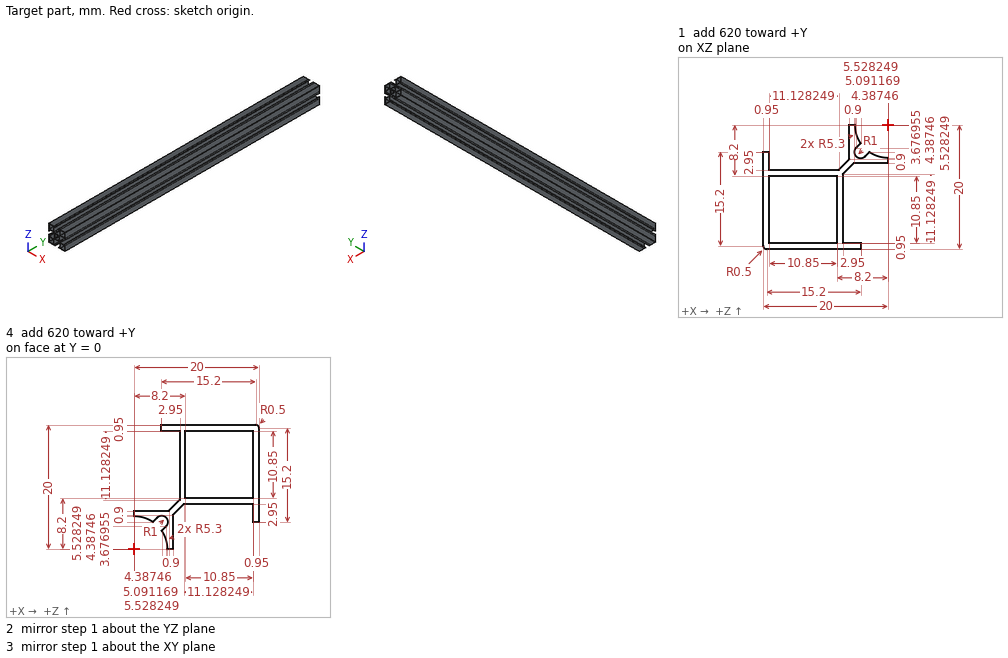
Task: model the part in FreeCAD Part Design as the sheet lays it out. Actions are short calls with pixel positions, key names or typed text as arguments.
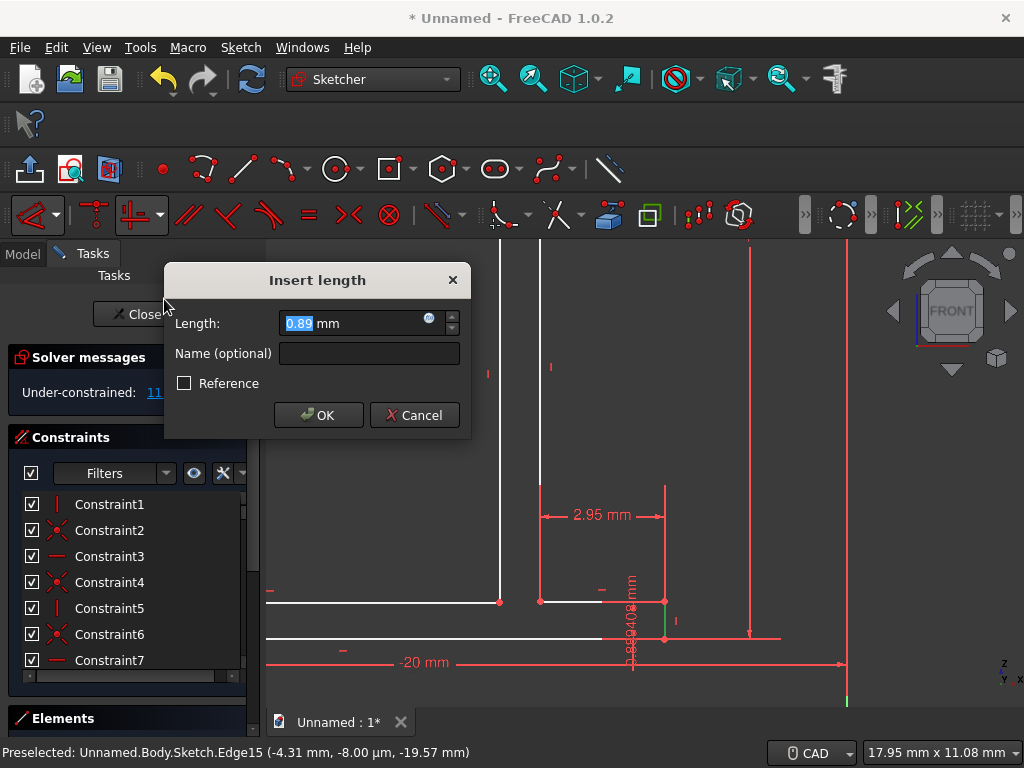
text(0.95)
key(Return)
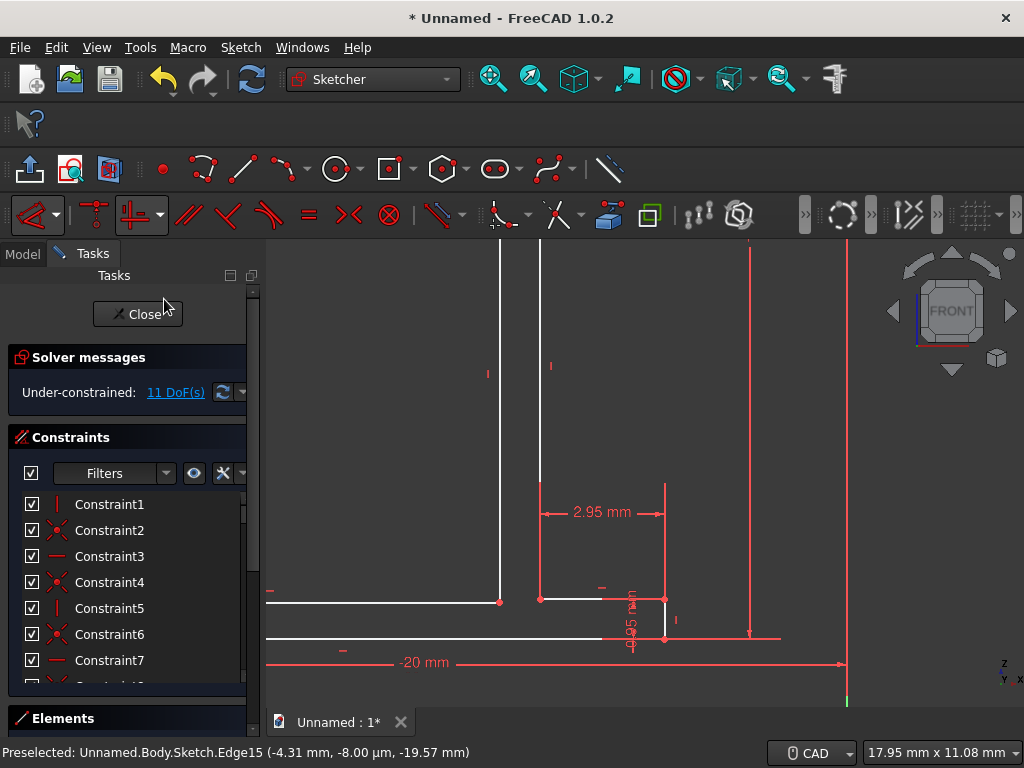
click(472, 639)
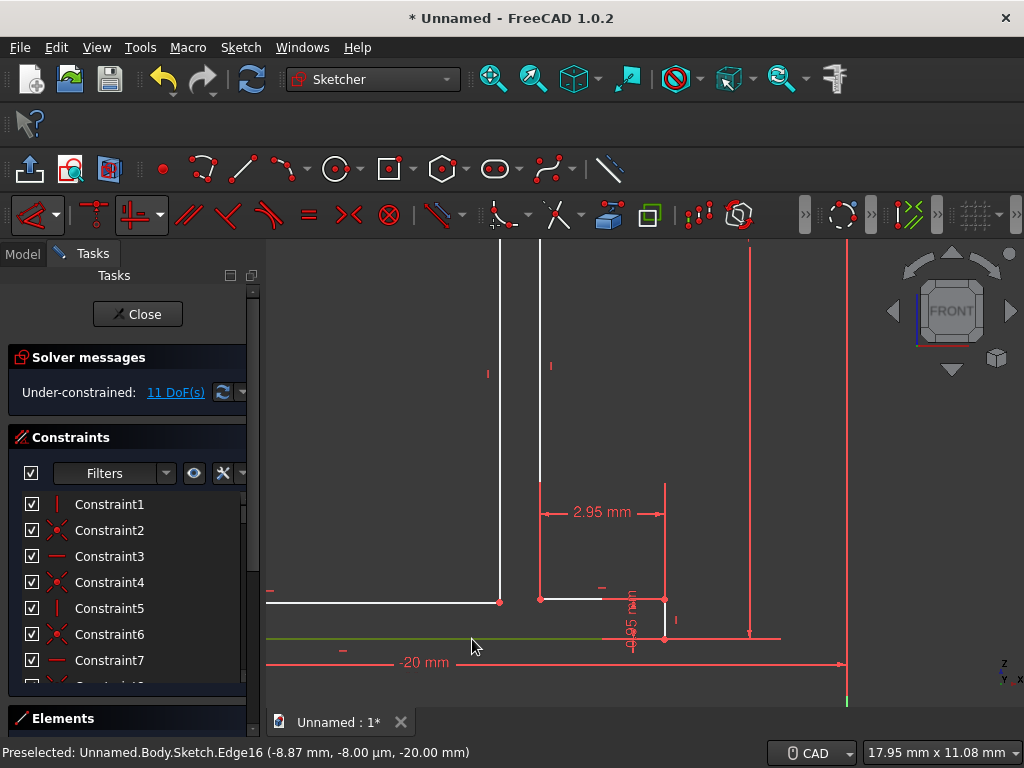
click(58, 216)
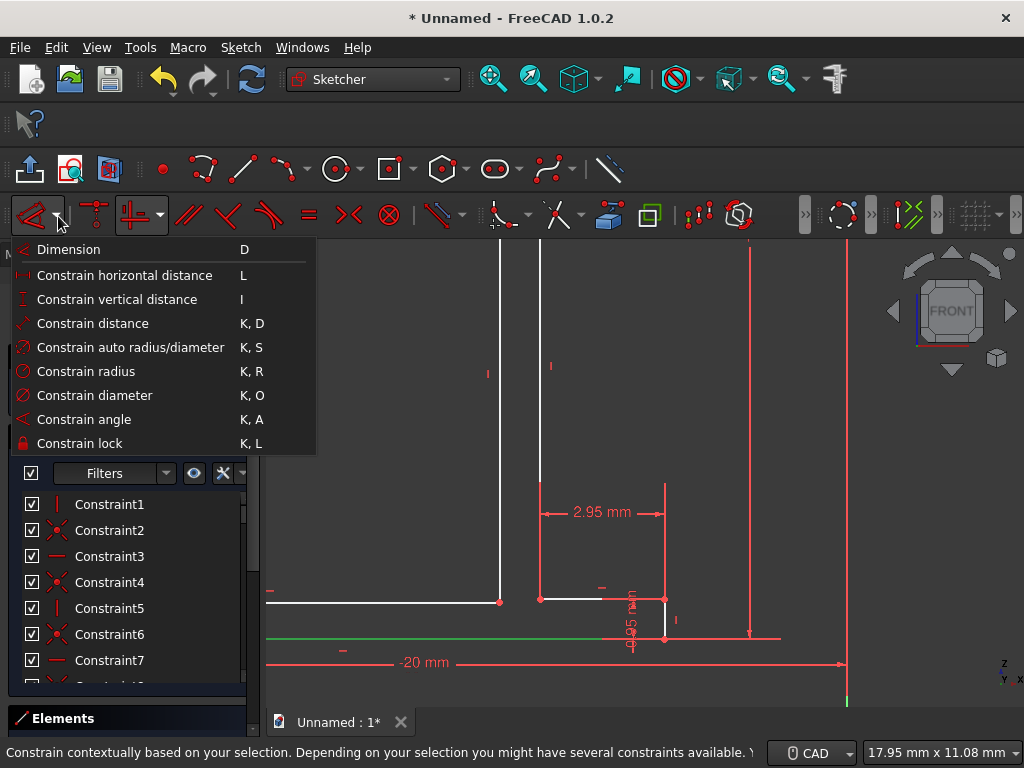
click(164, 275)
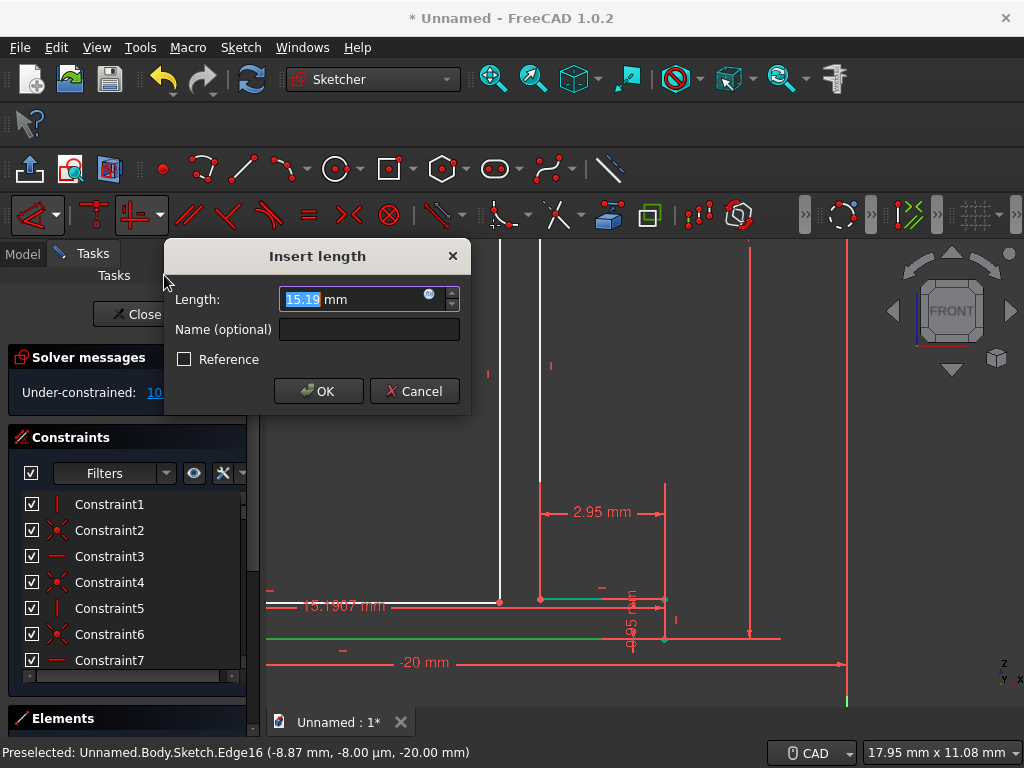
text(15.2)
key(Return)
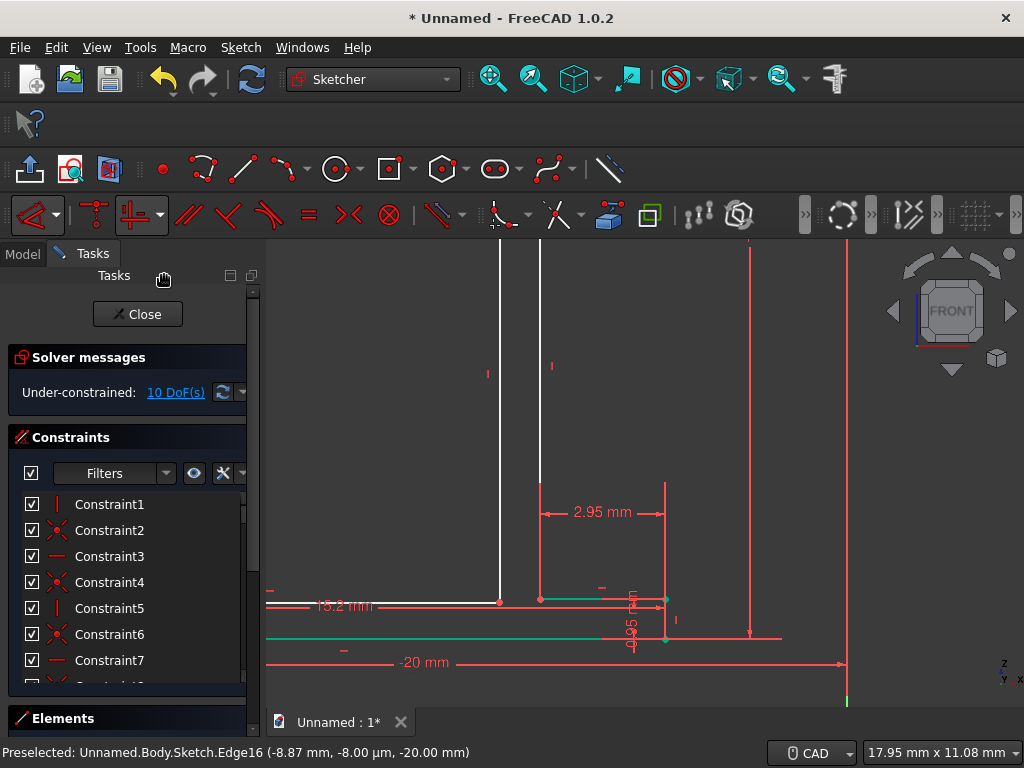
scroll(665, 622, down, 5)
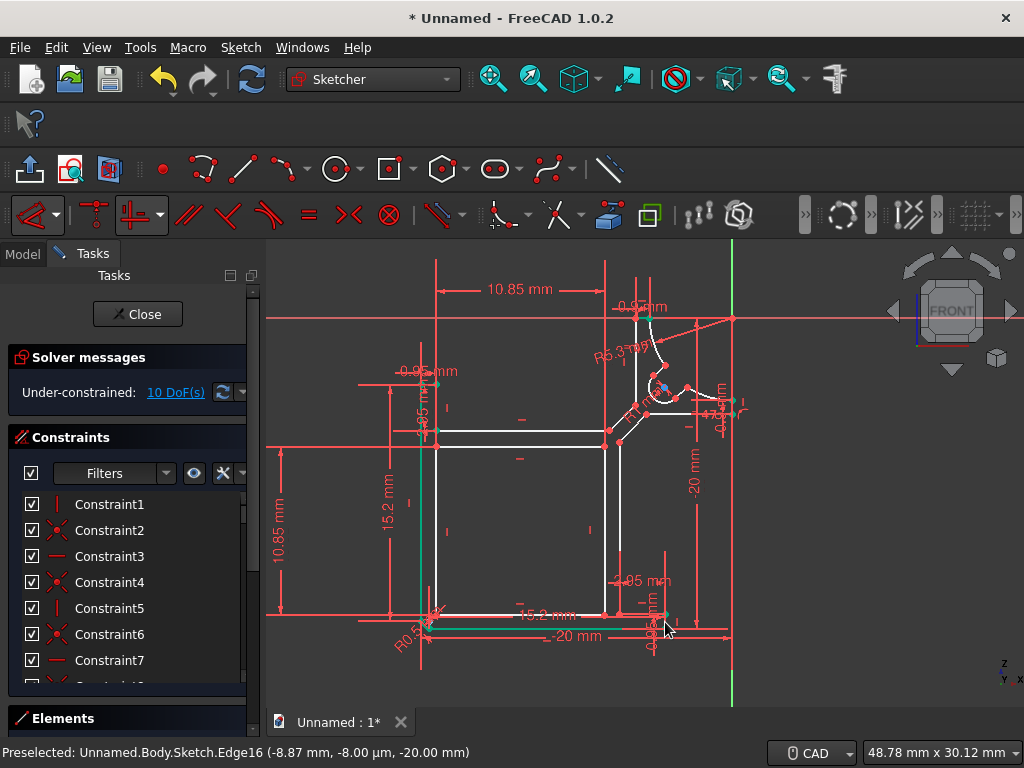
click(436, 447)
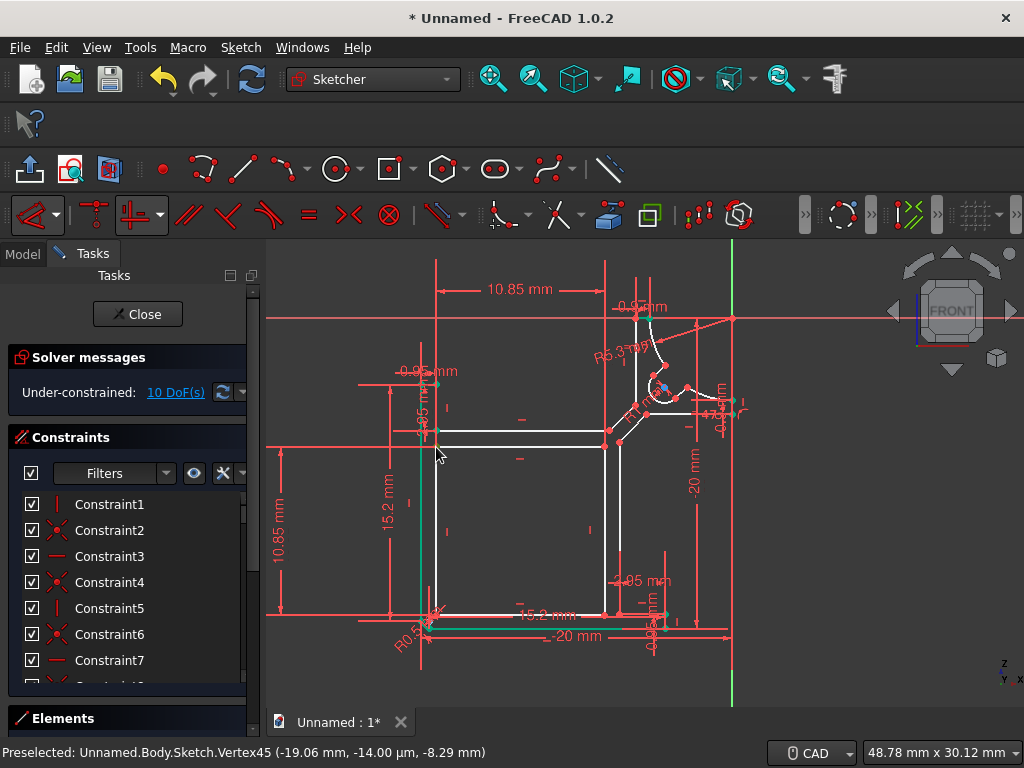
click(58, 216)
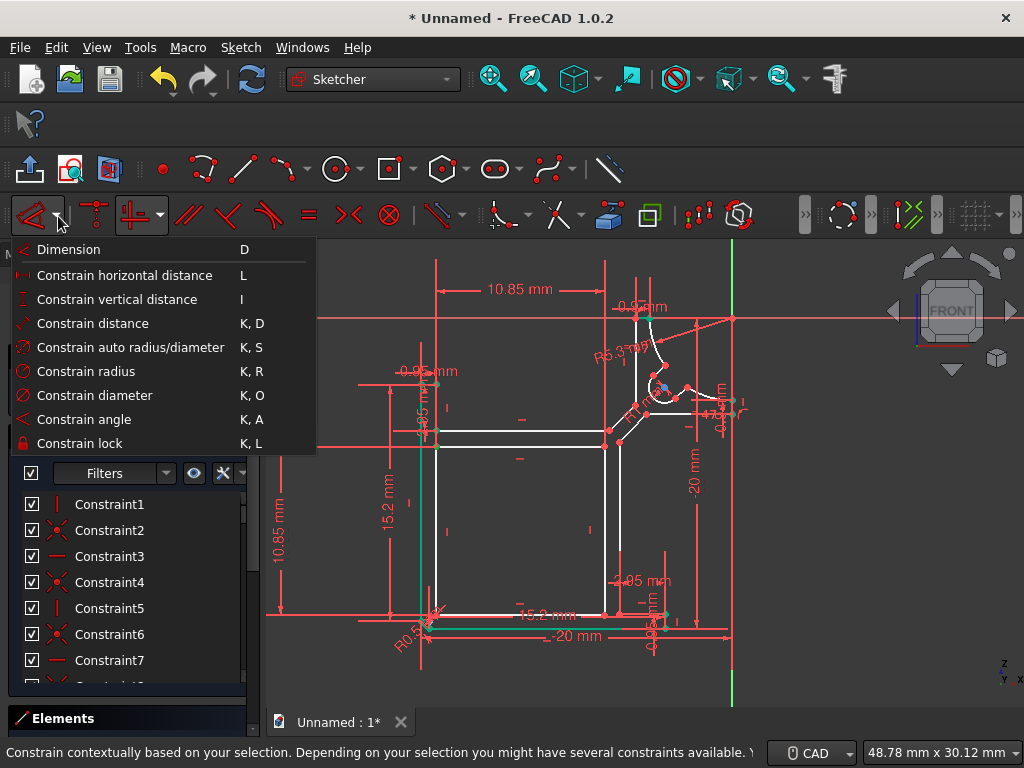
click(164, 299)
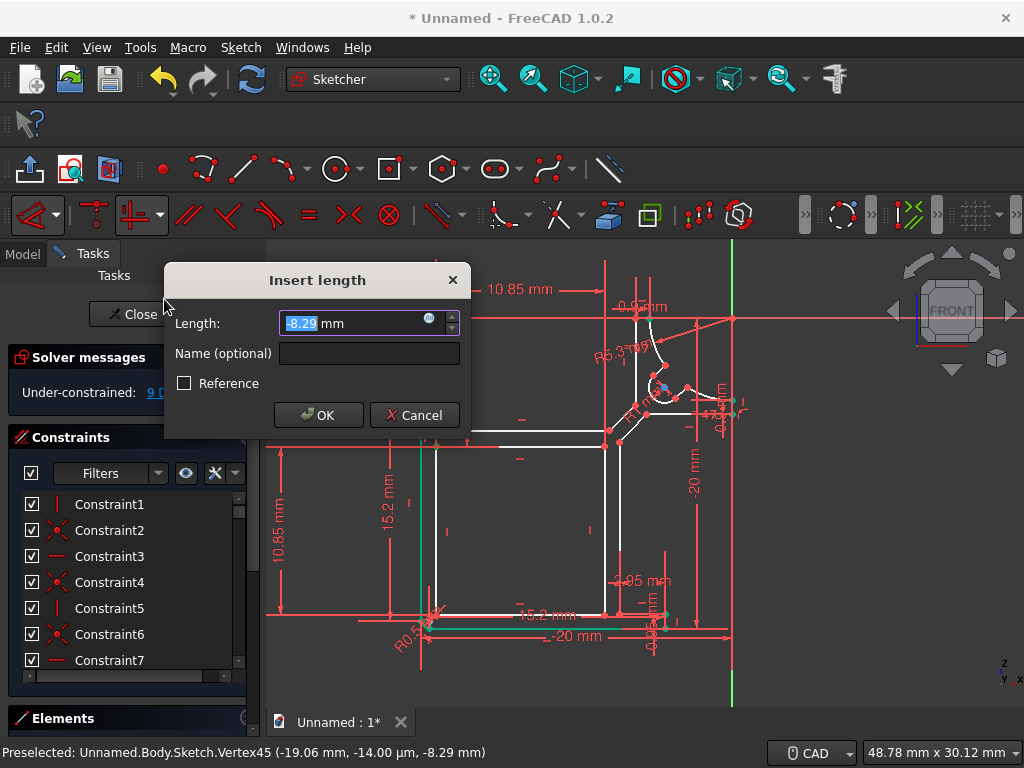
text(-8.2)
key(Return)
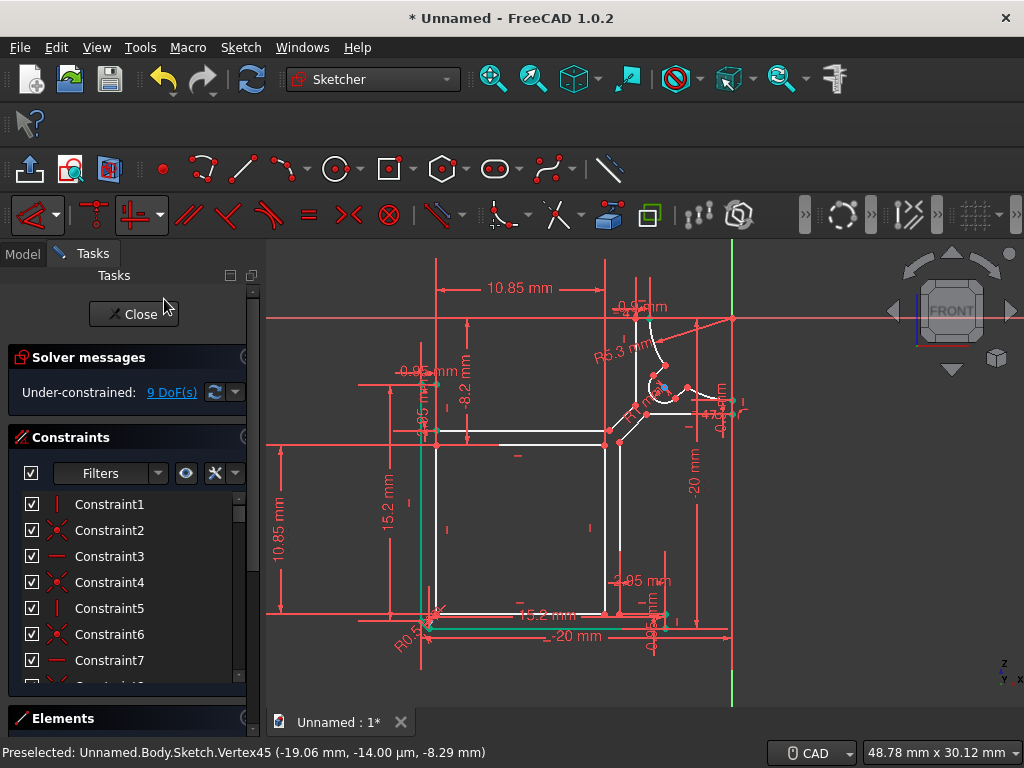
click(605, 614)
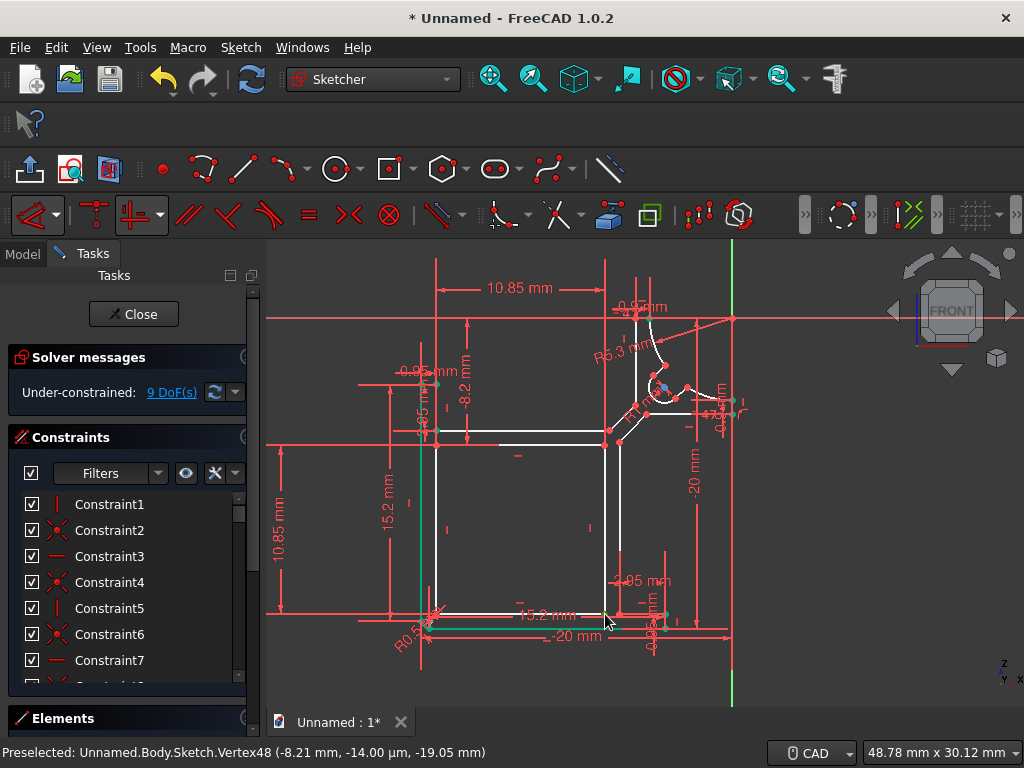
key(l)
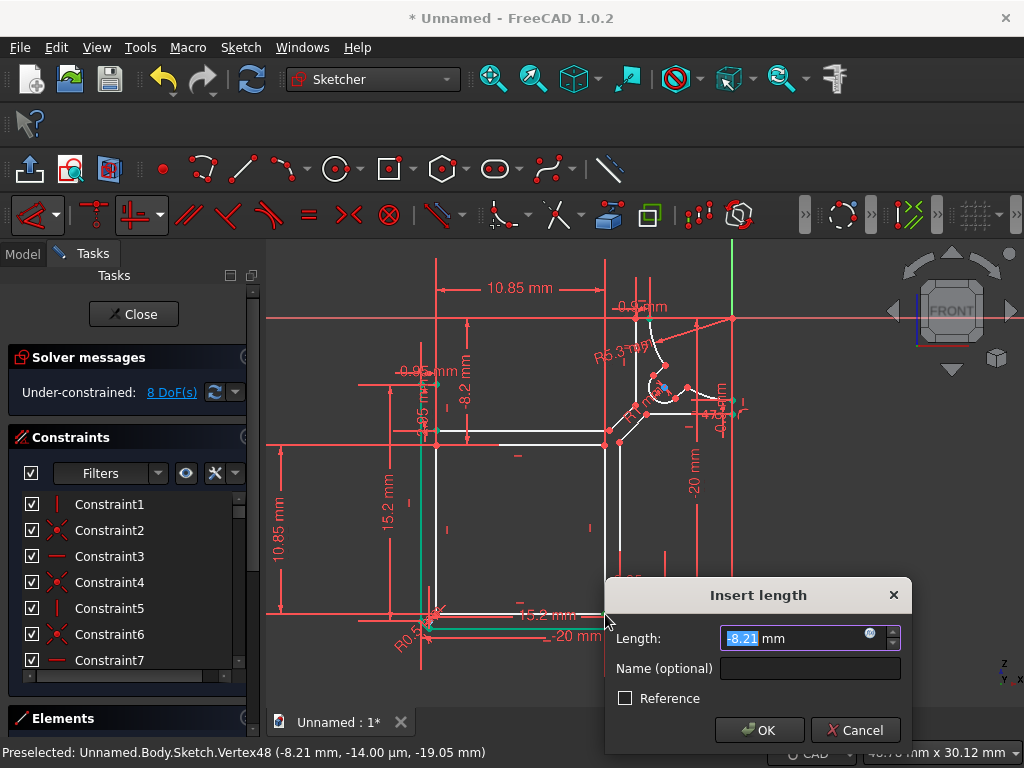
text(-8.2)
key(Return)